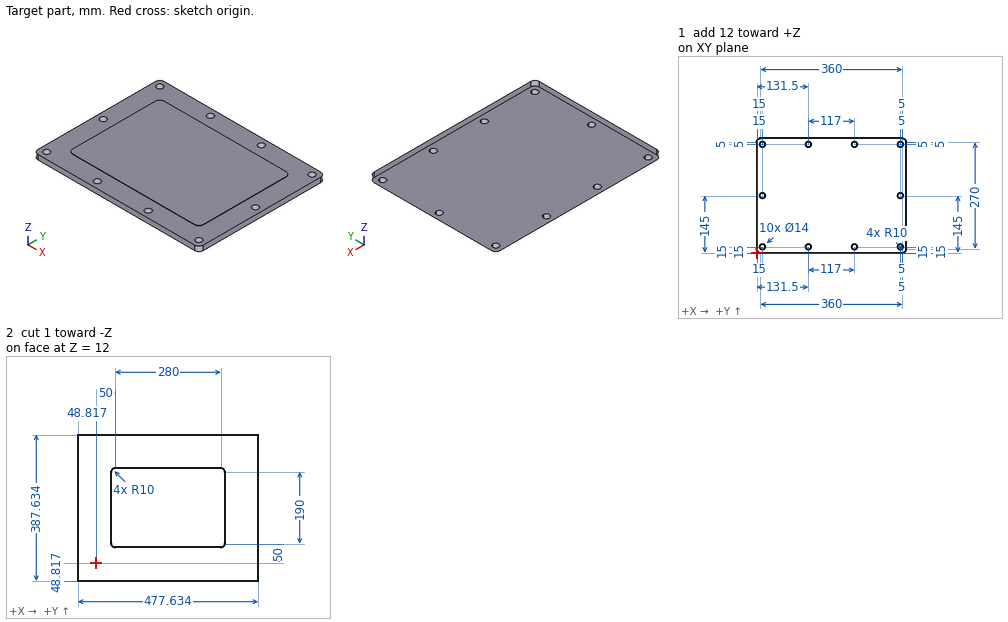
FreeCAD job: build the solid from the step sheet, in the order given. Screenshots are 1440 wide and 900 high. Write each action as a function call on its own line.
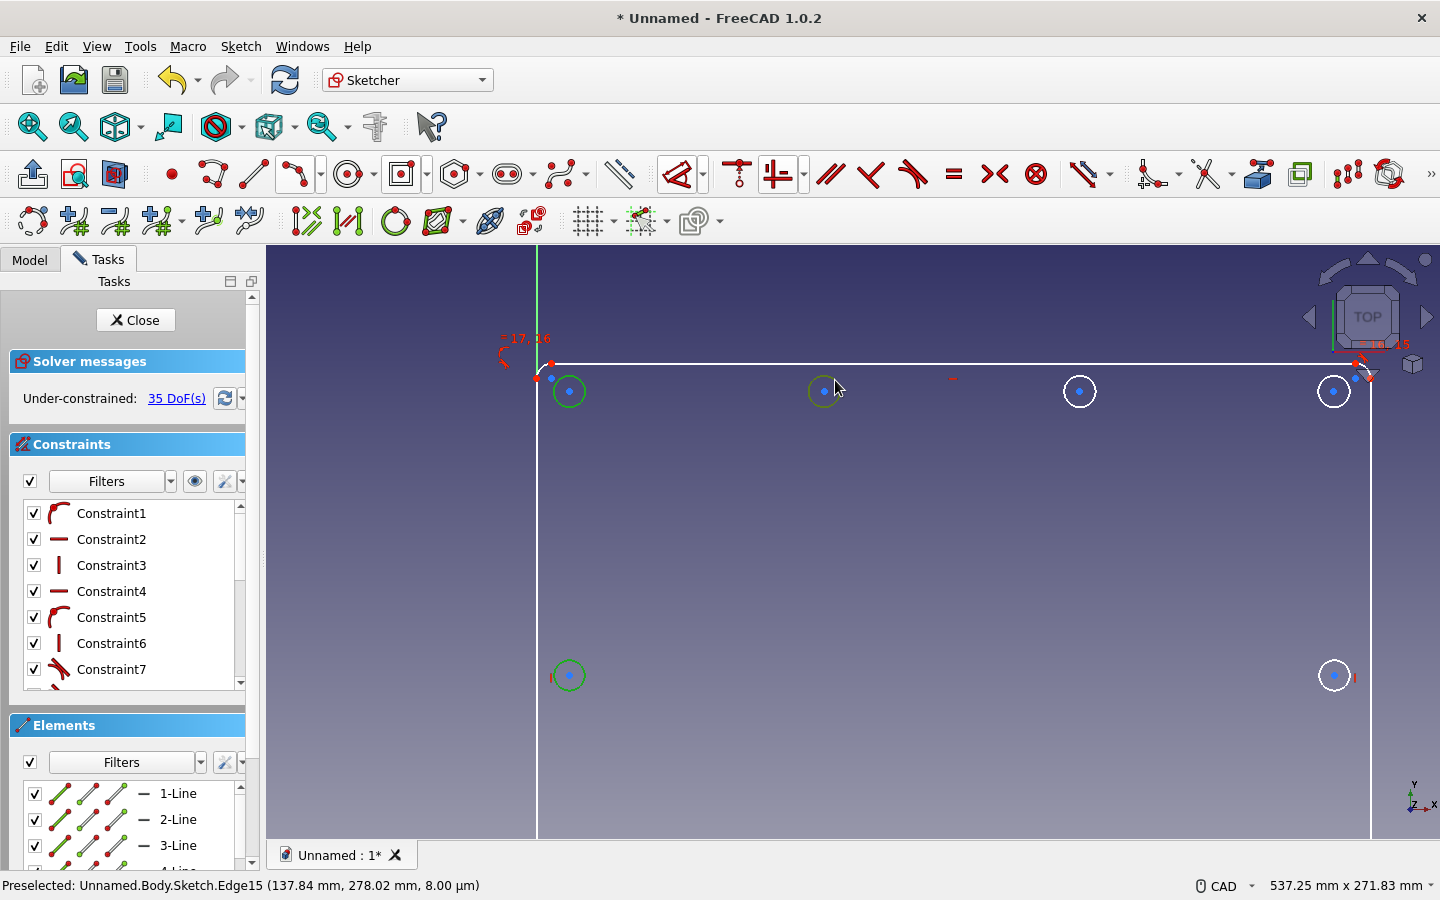
scroll(581, 381, down, 3)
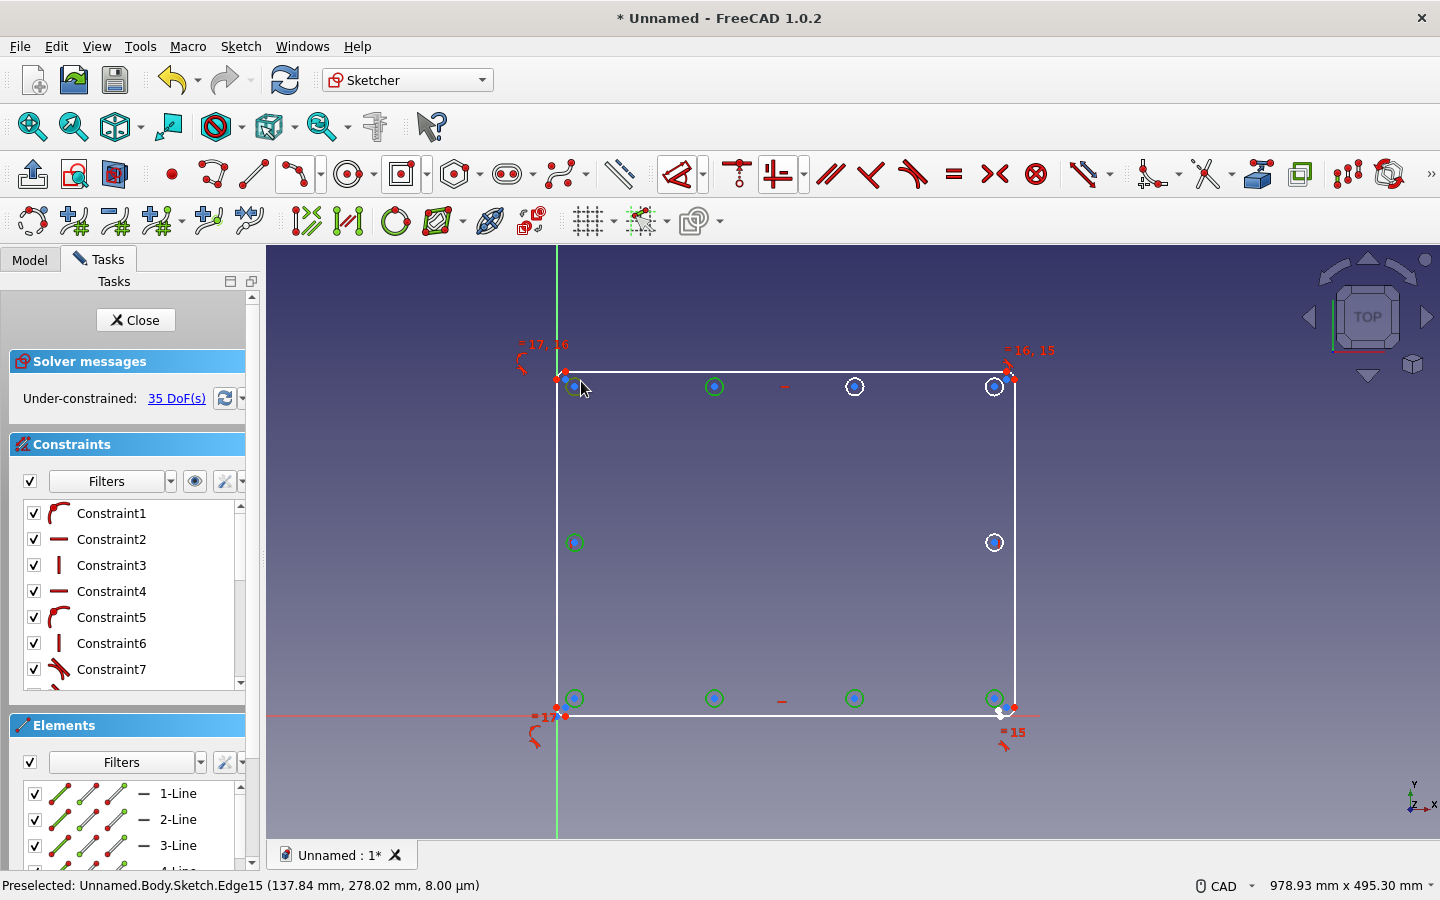
scroll(1001, 537, up, 3)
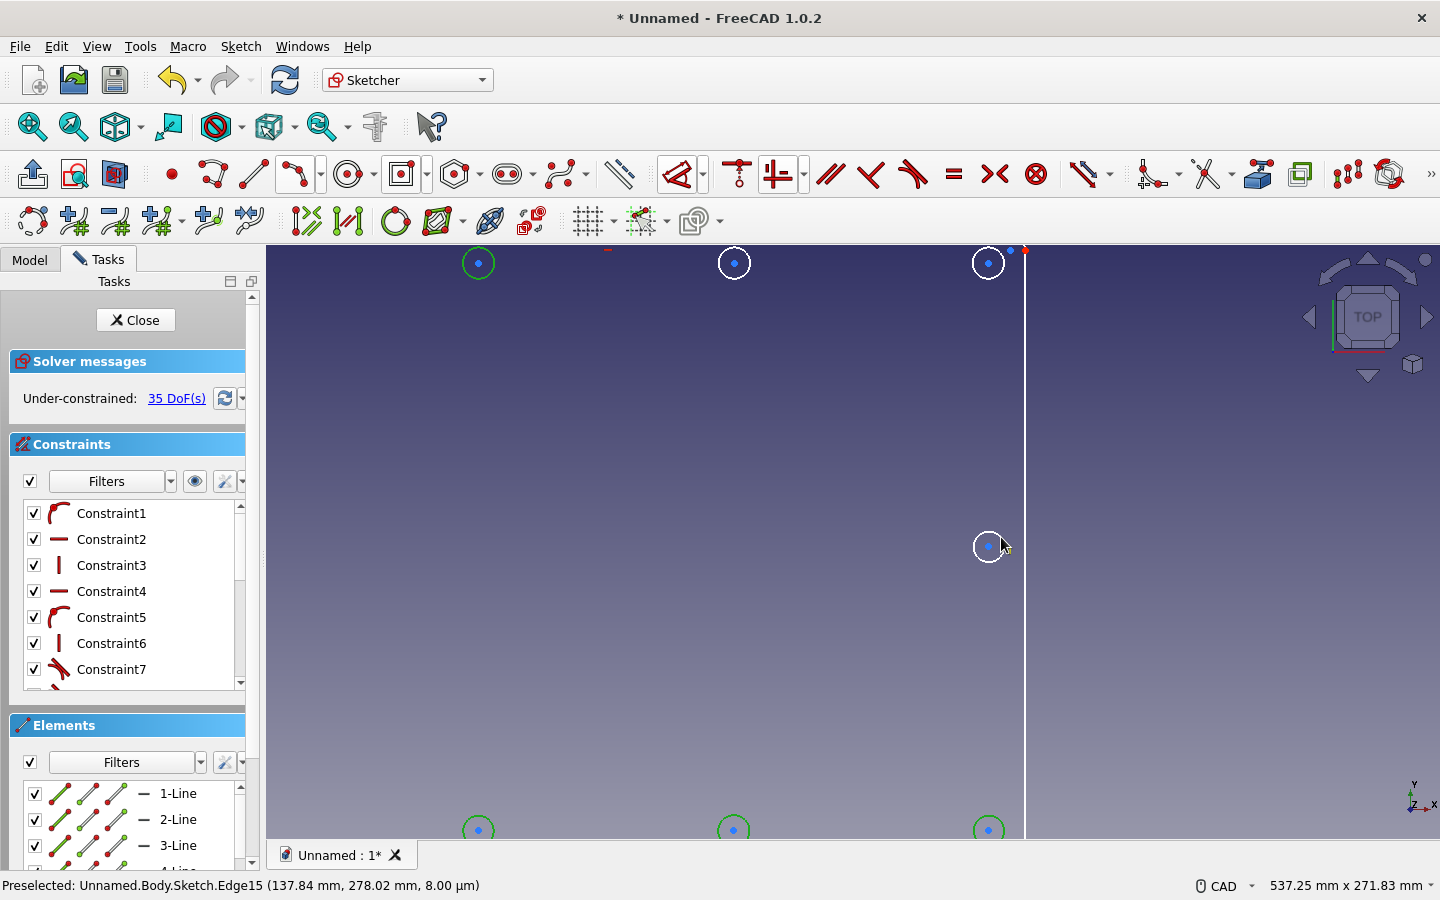
click(1000, 536)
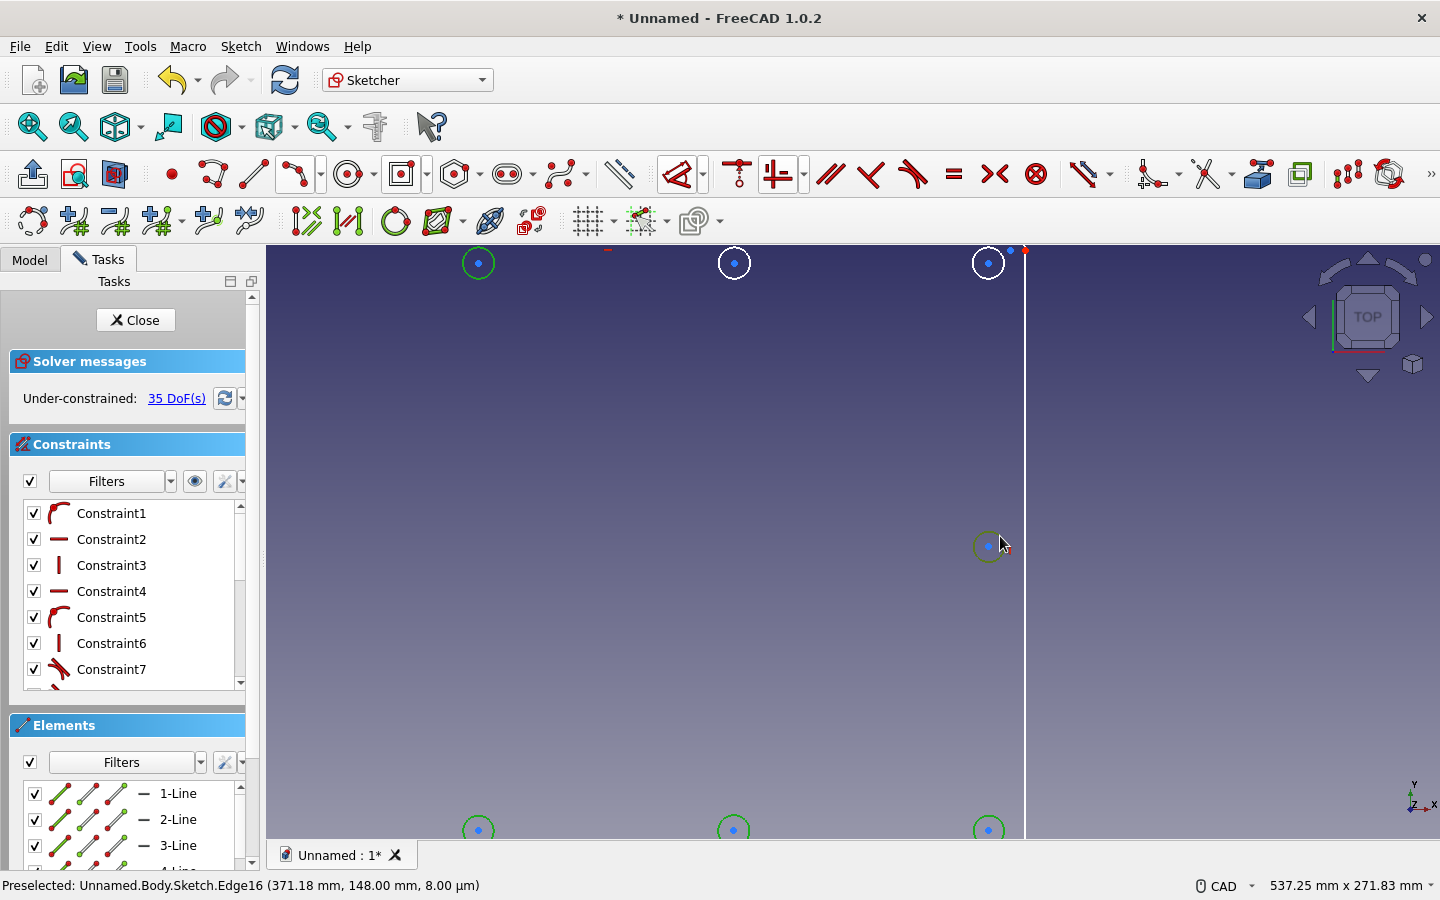
click(723, 274)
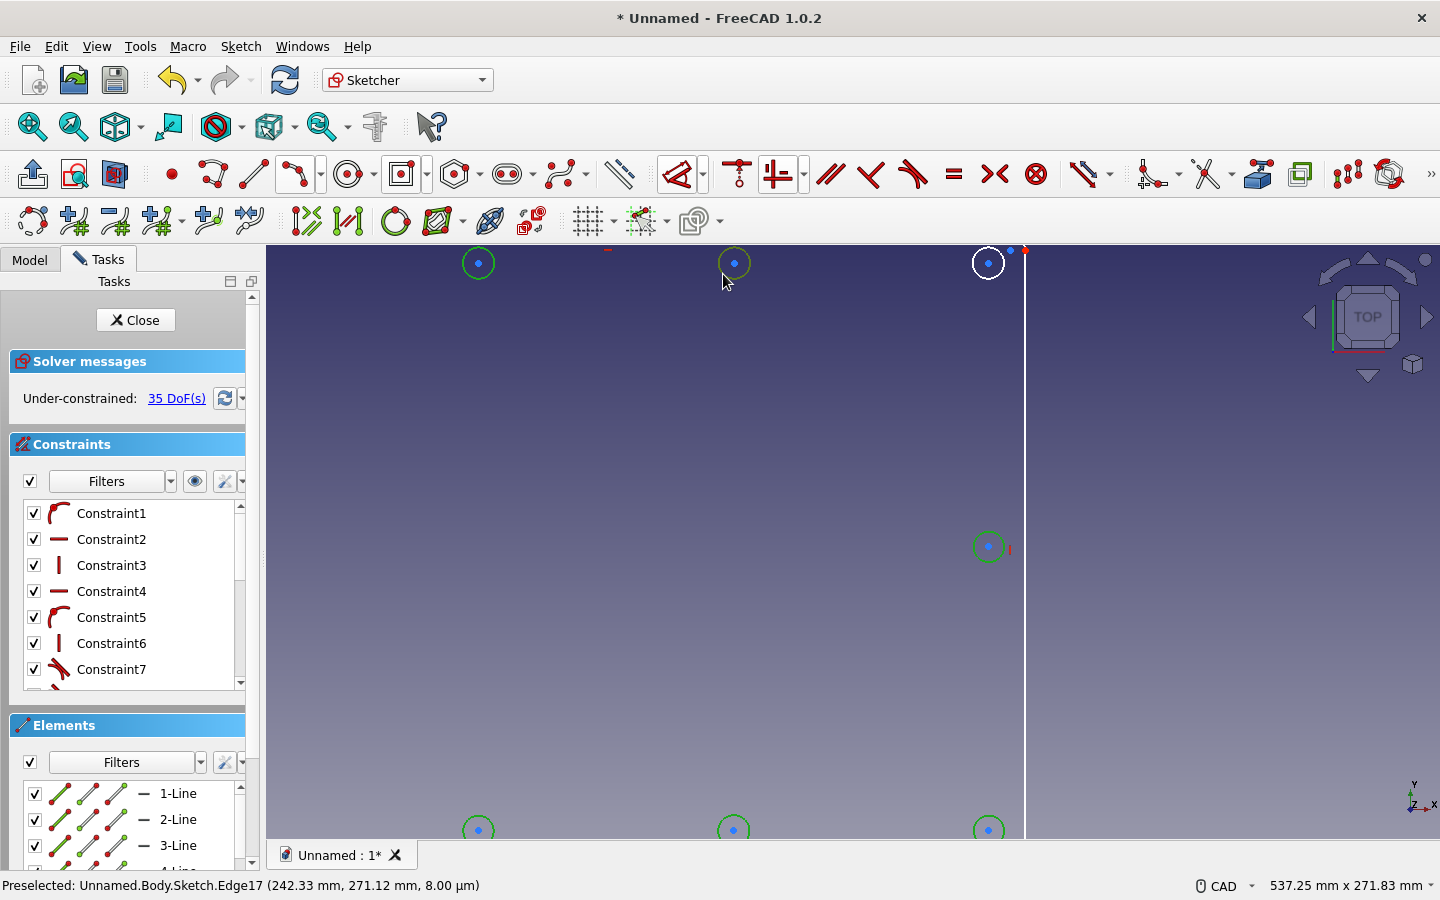
click(977, 274)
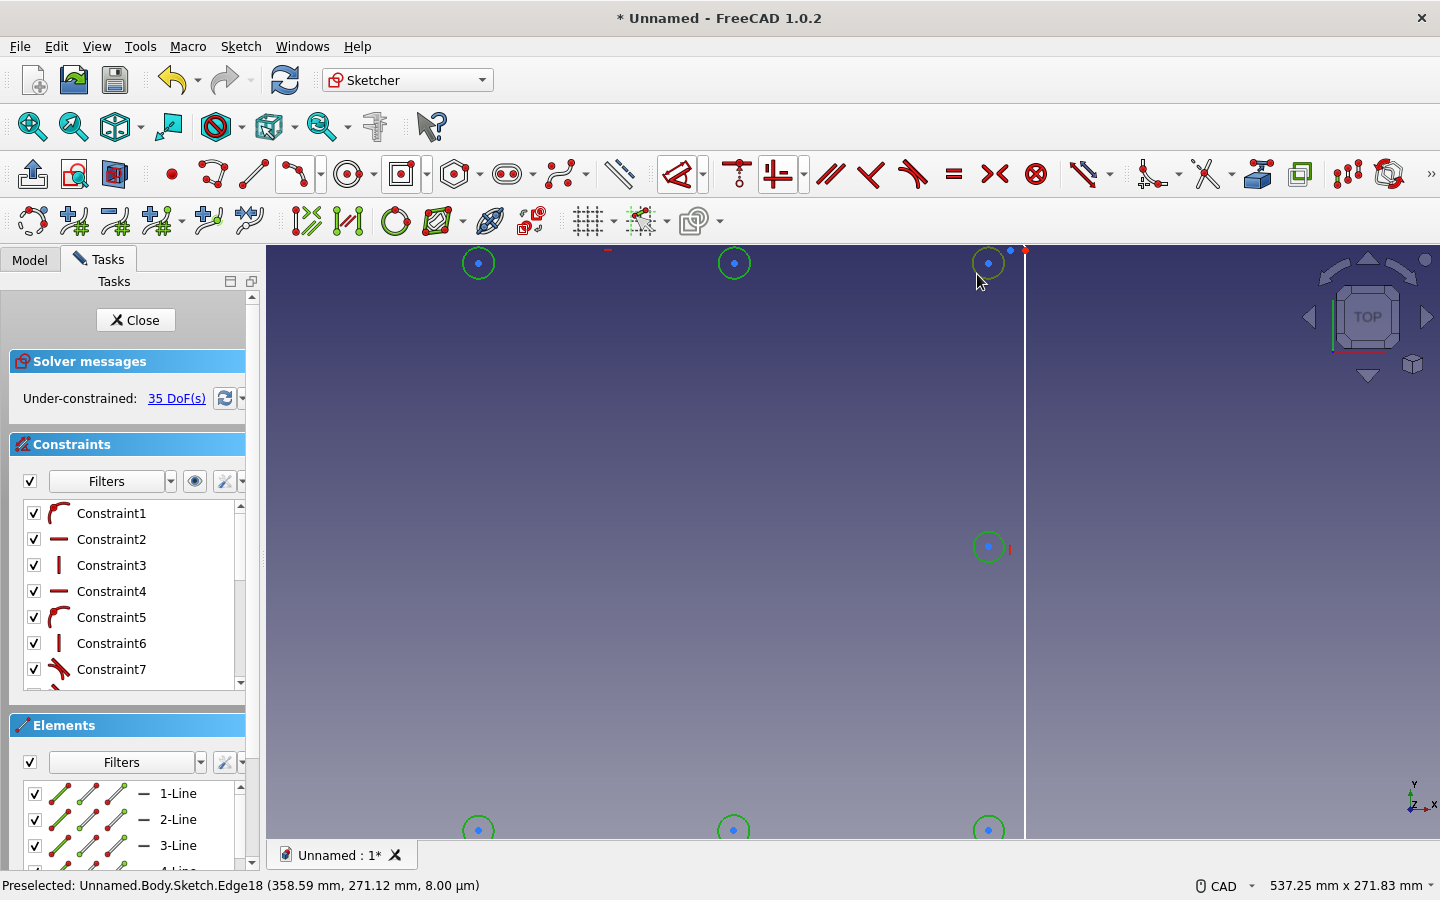
click(954, 174)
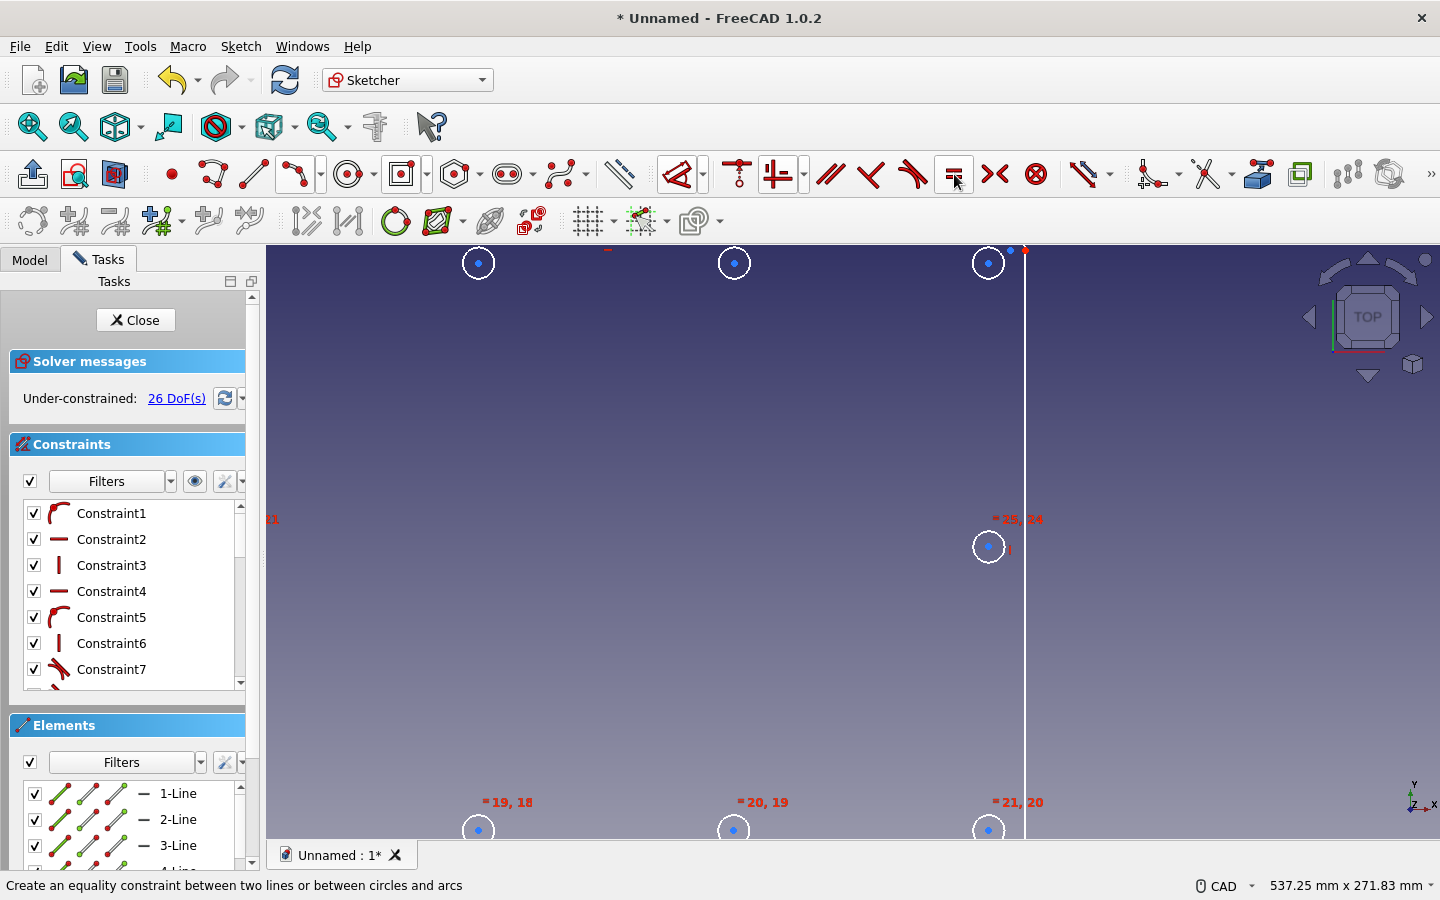
scroll(1001, 537, down, 3)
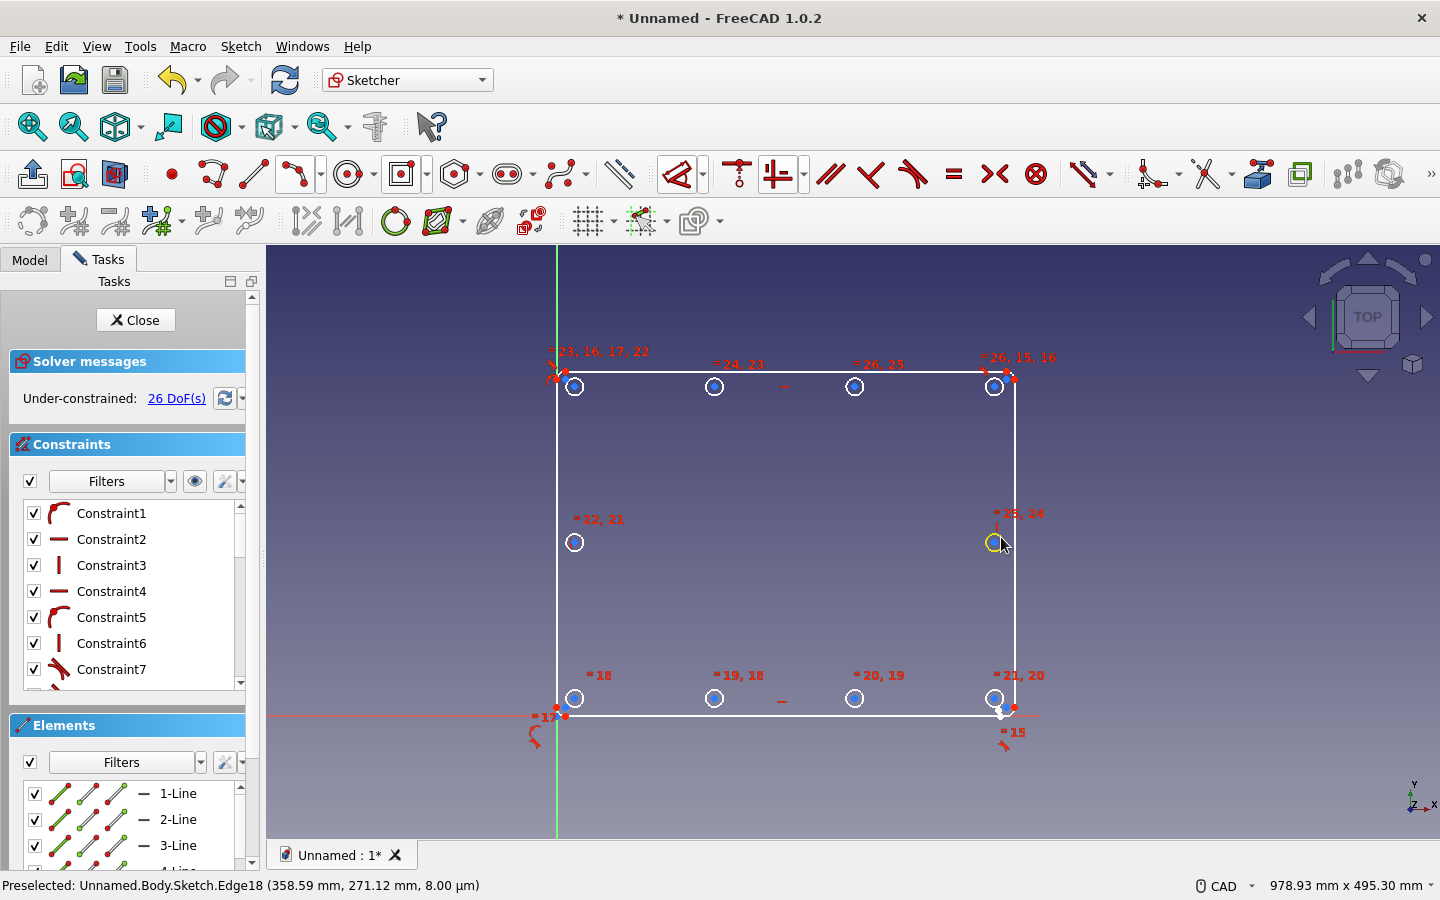
scroll(1012, 714, up, 6)